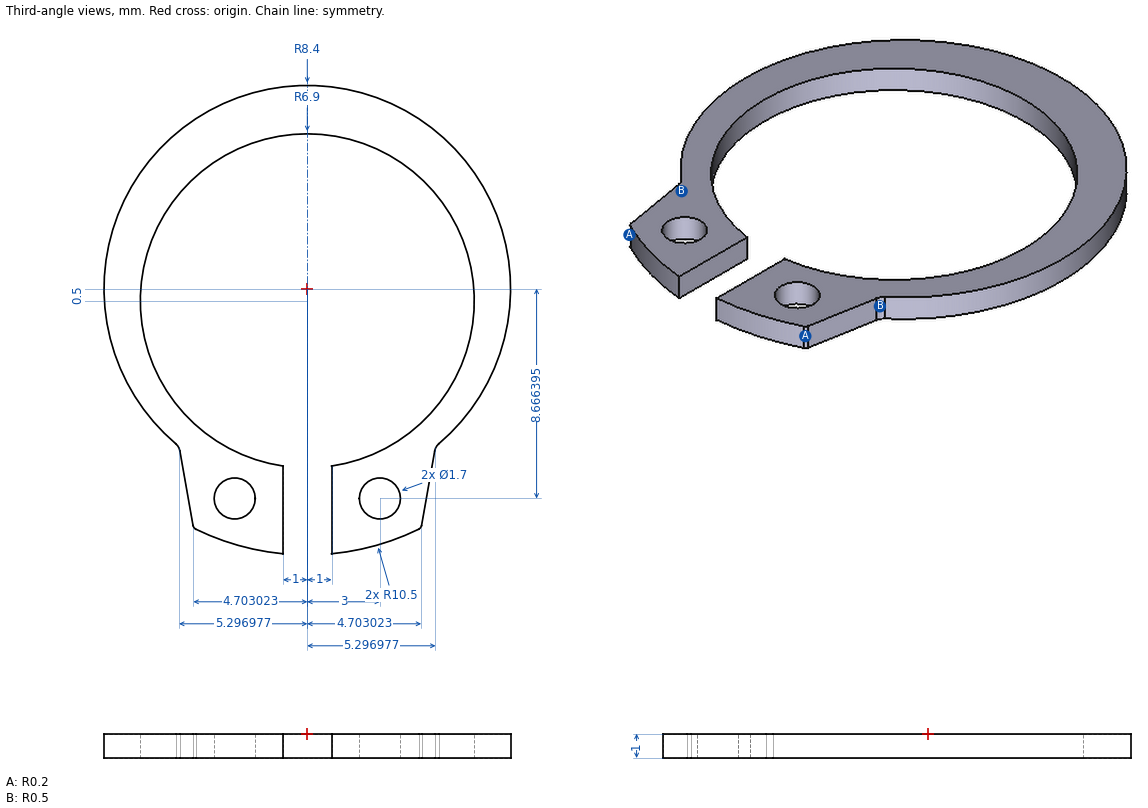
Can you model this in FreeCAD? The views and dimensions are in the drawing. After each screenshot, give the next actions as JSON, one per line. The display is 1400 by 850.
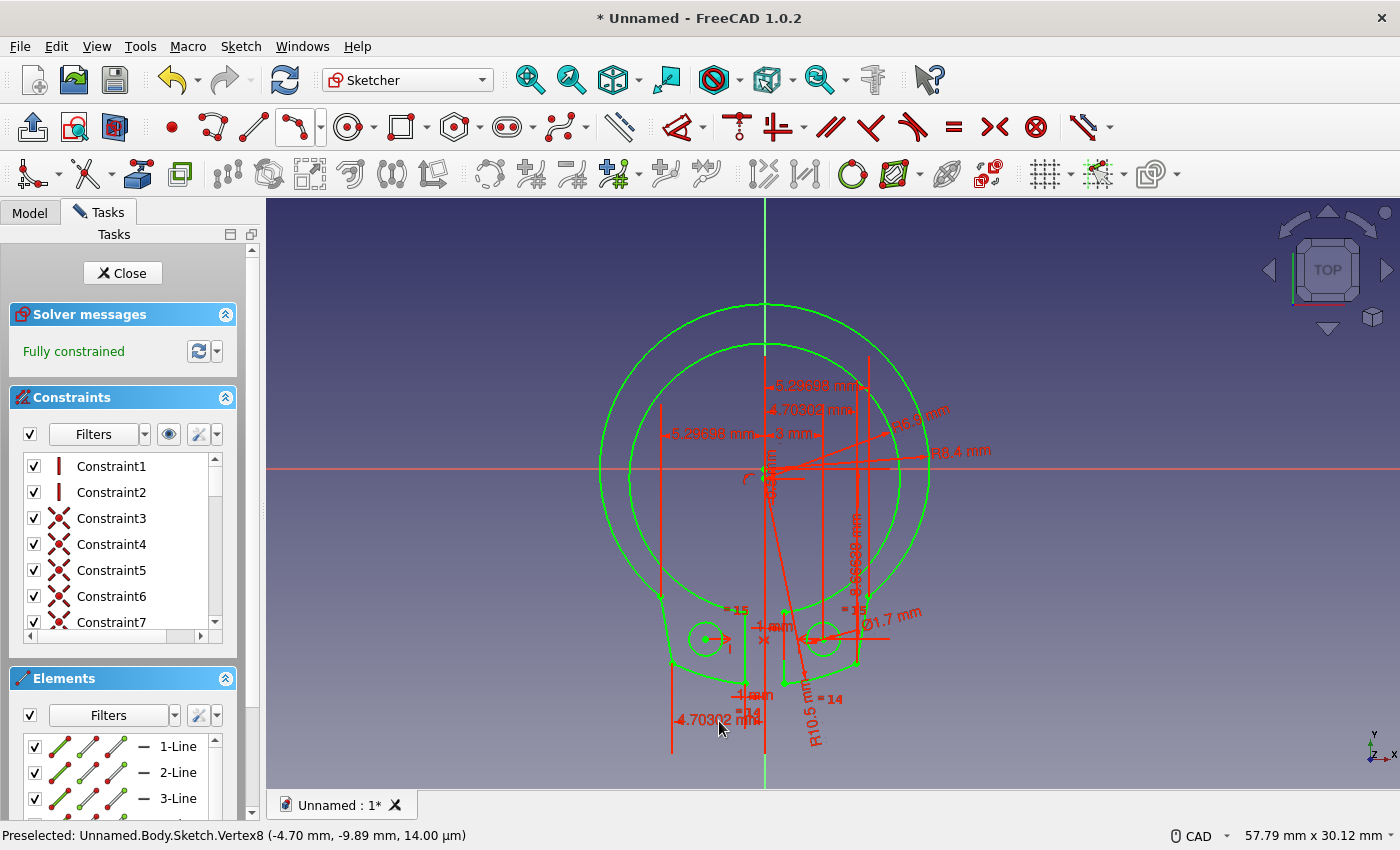
{"action": "left_click", "coordinate": [123, 273]}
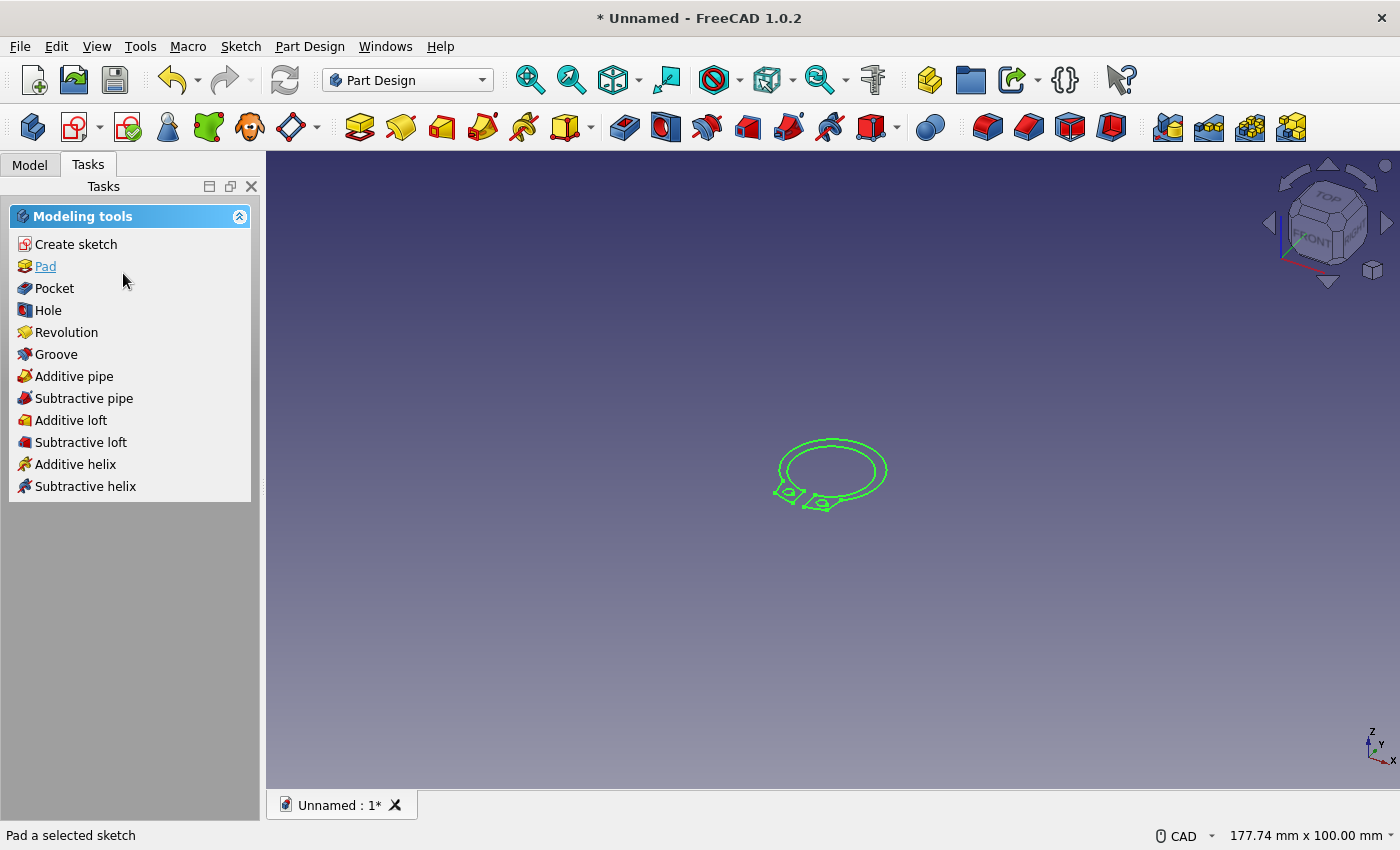
{"action": "left_click", "coordinate": [360, 128]}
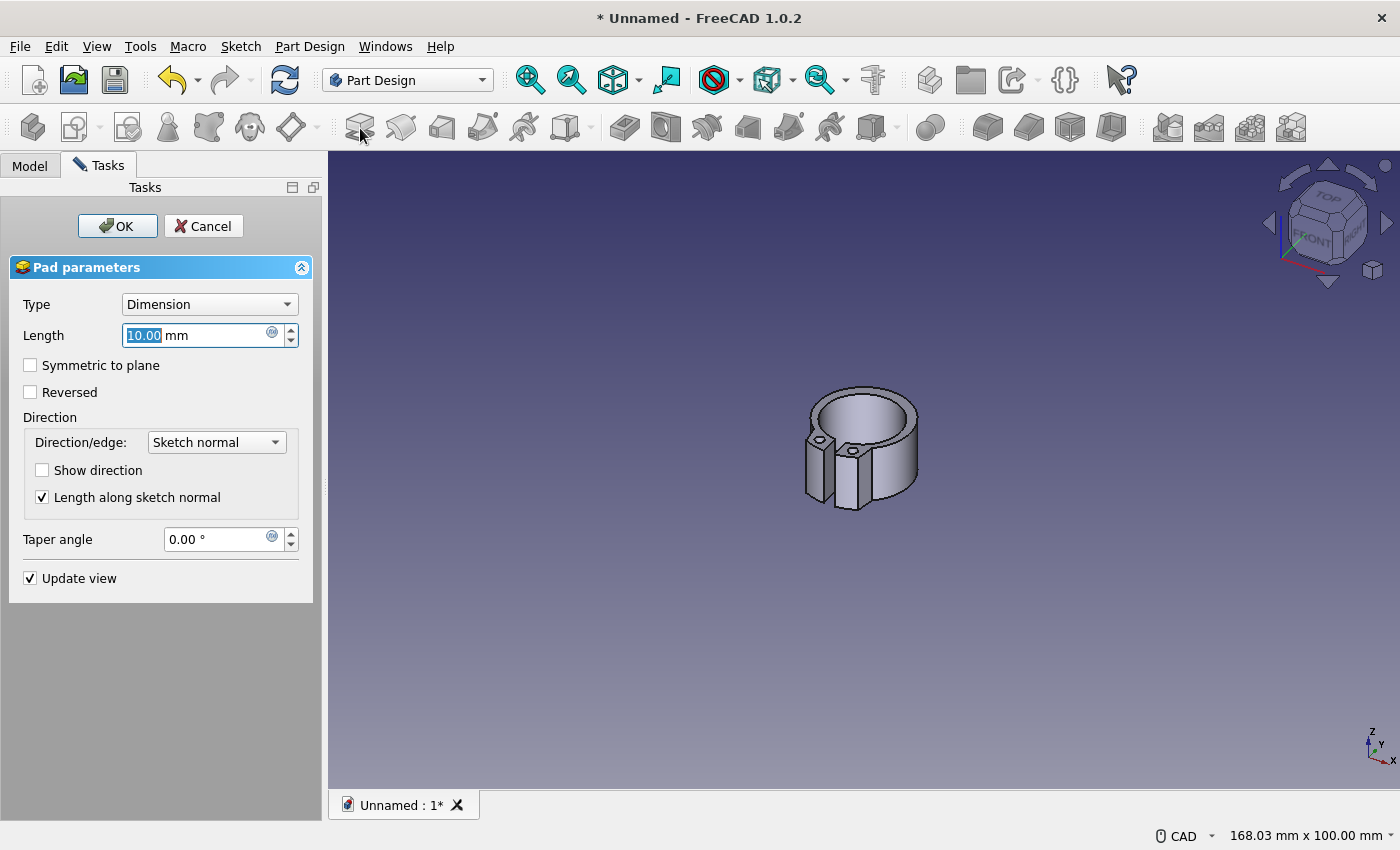
{"action": "type", "text": "1"}
{"action": "key", "text": "Tab"}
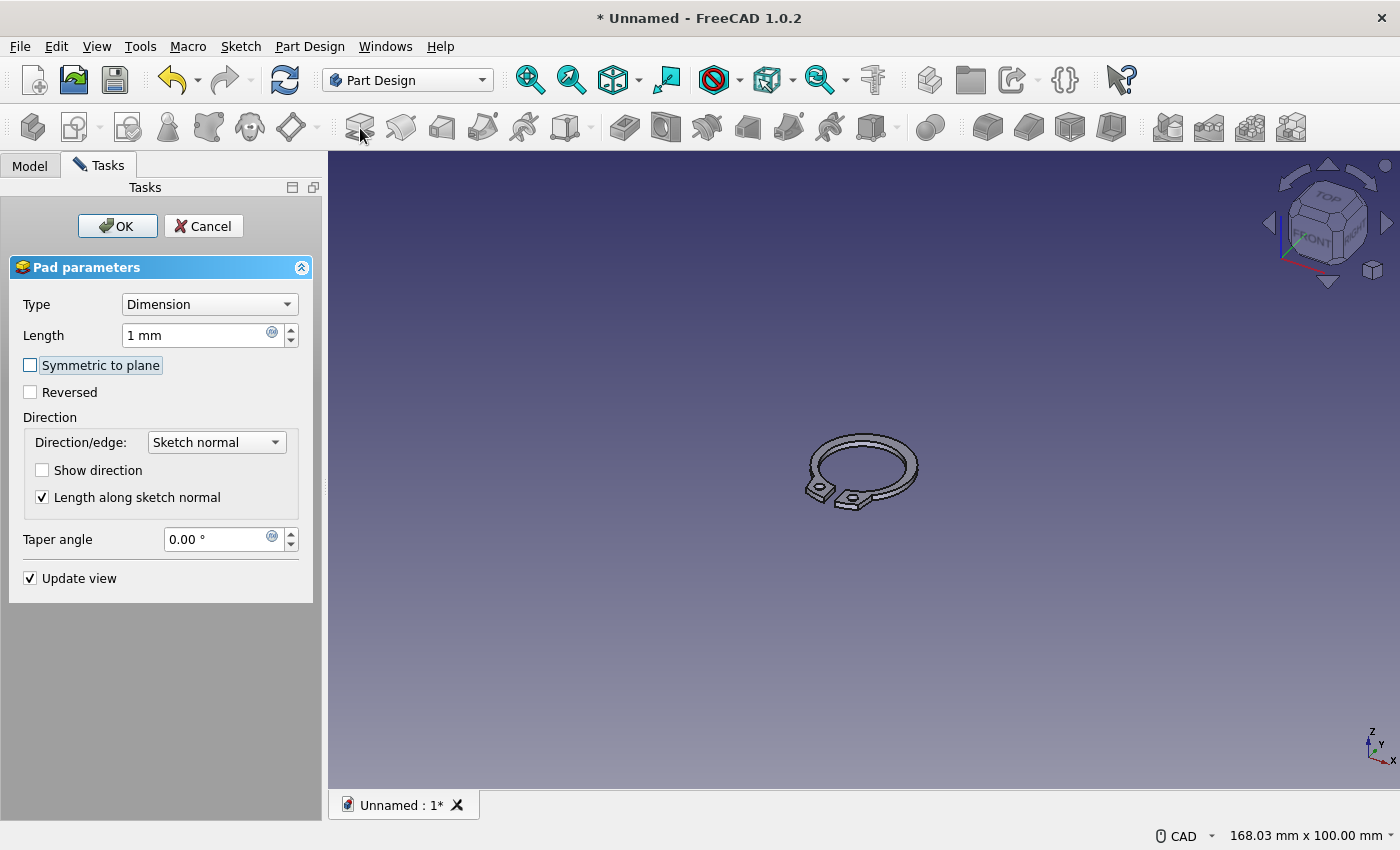
{"action": "left_click", "coordinate": [31, 392]}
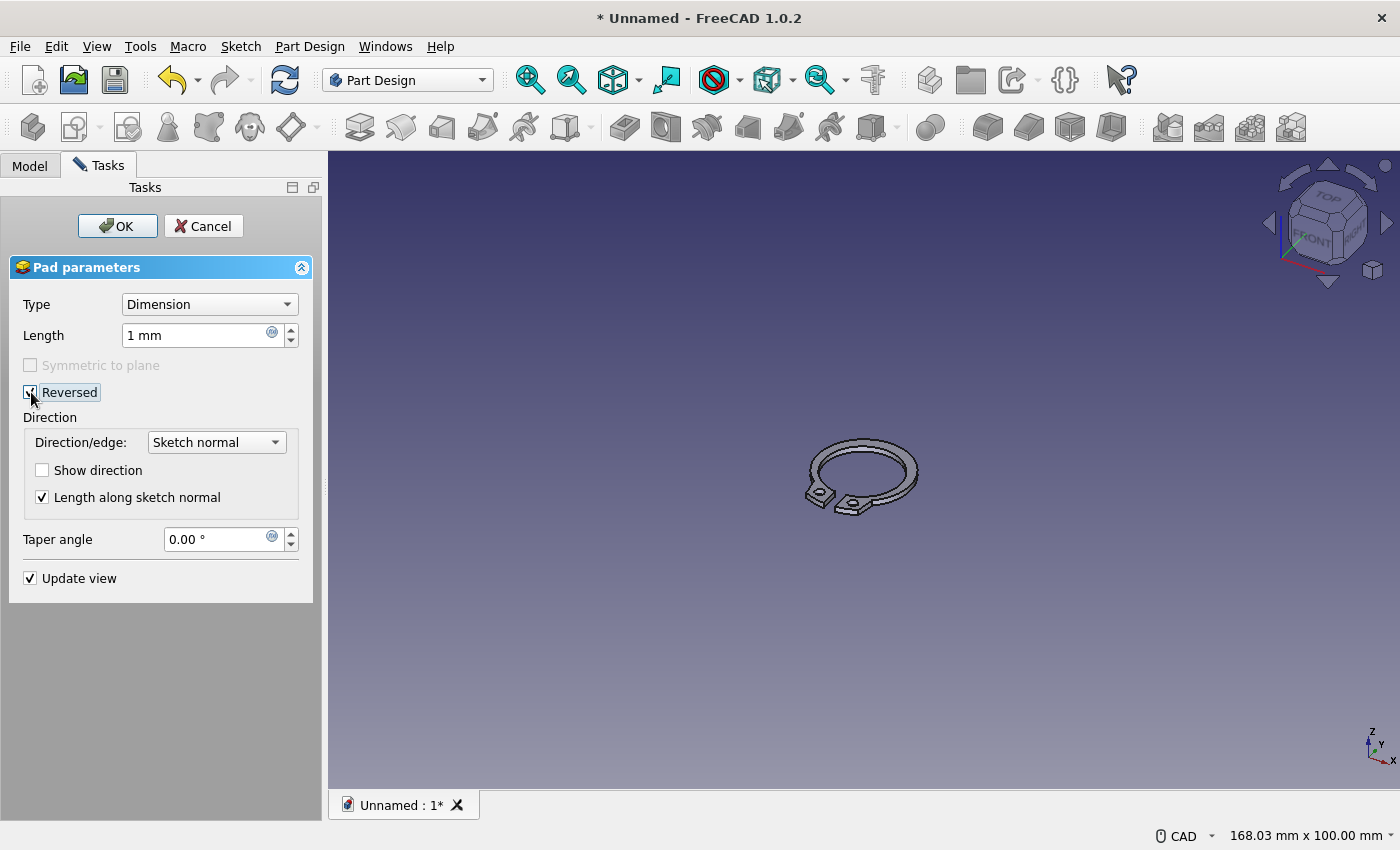
{"action": "left_click", "coordinate": [118, 226]}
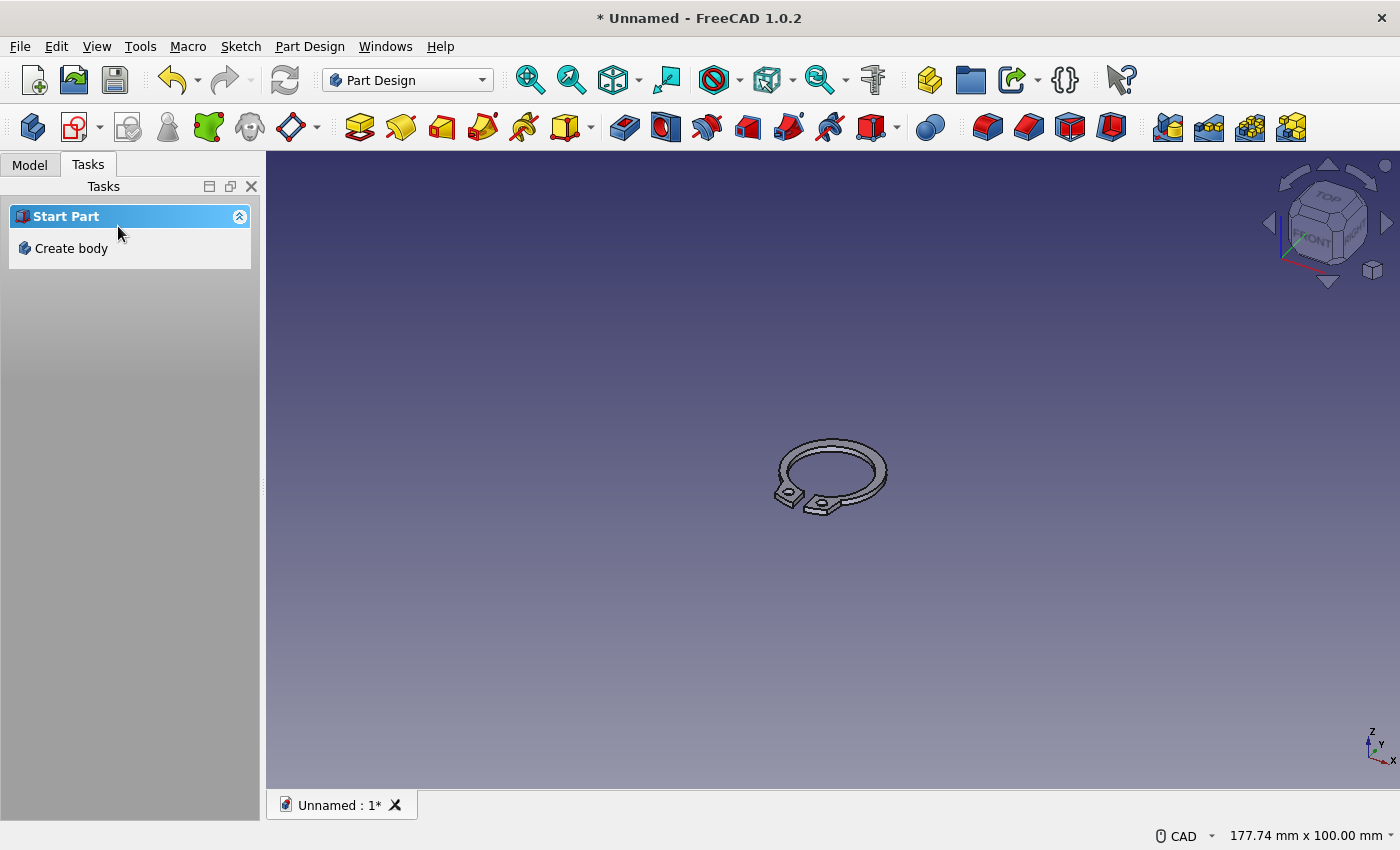
{"action": "left_click", "coordinate": [531, 80]}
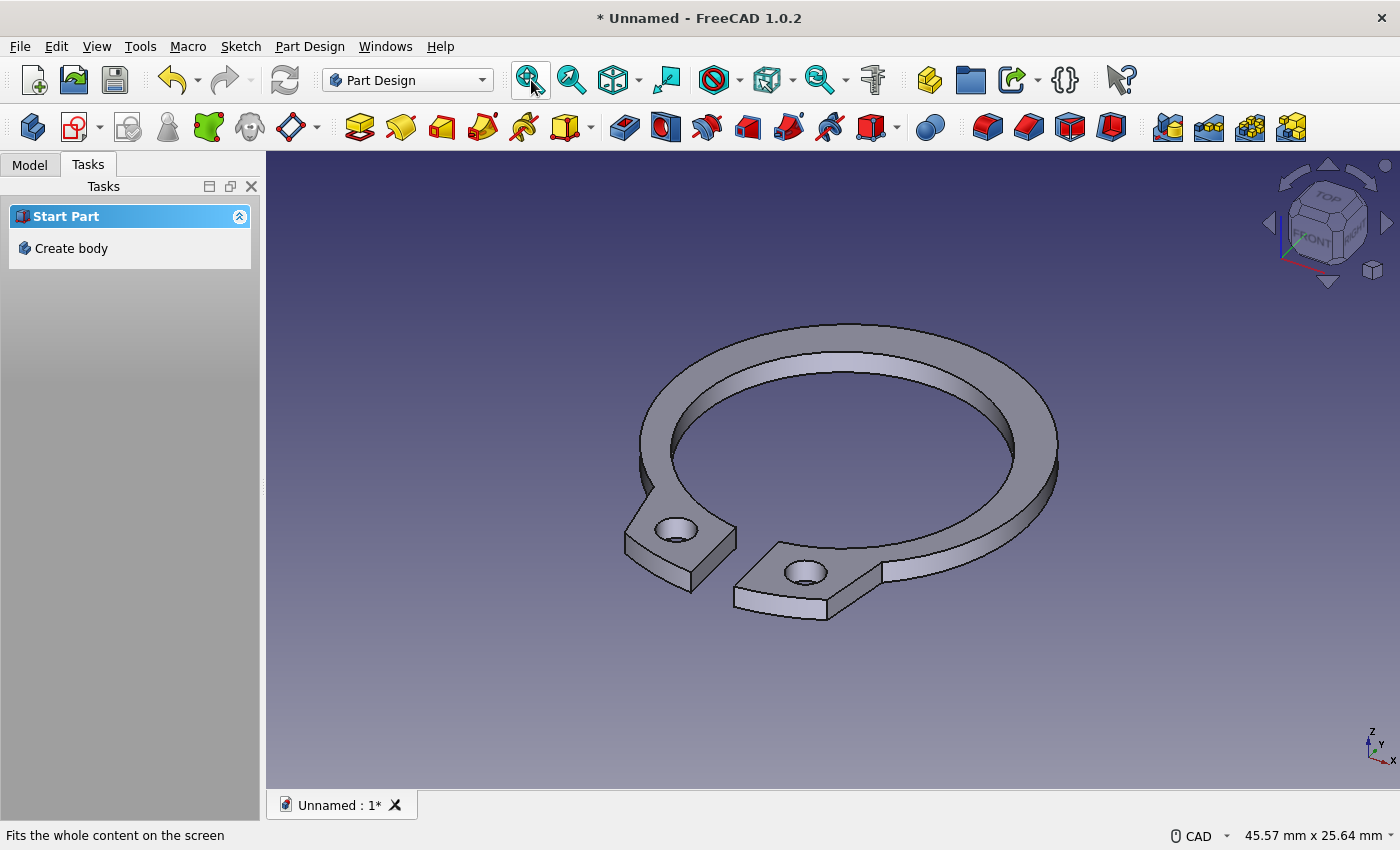
{"action": "left_click", "coordinate": [827, 609]}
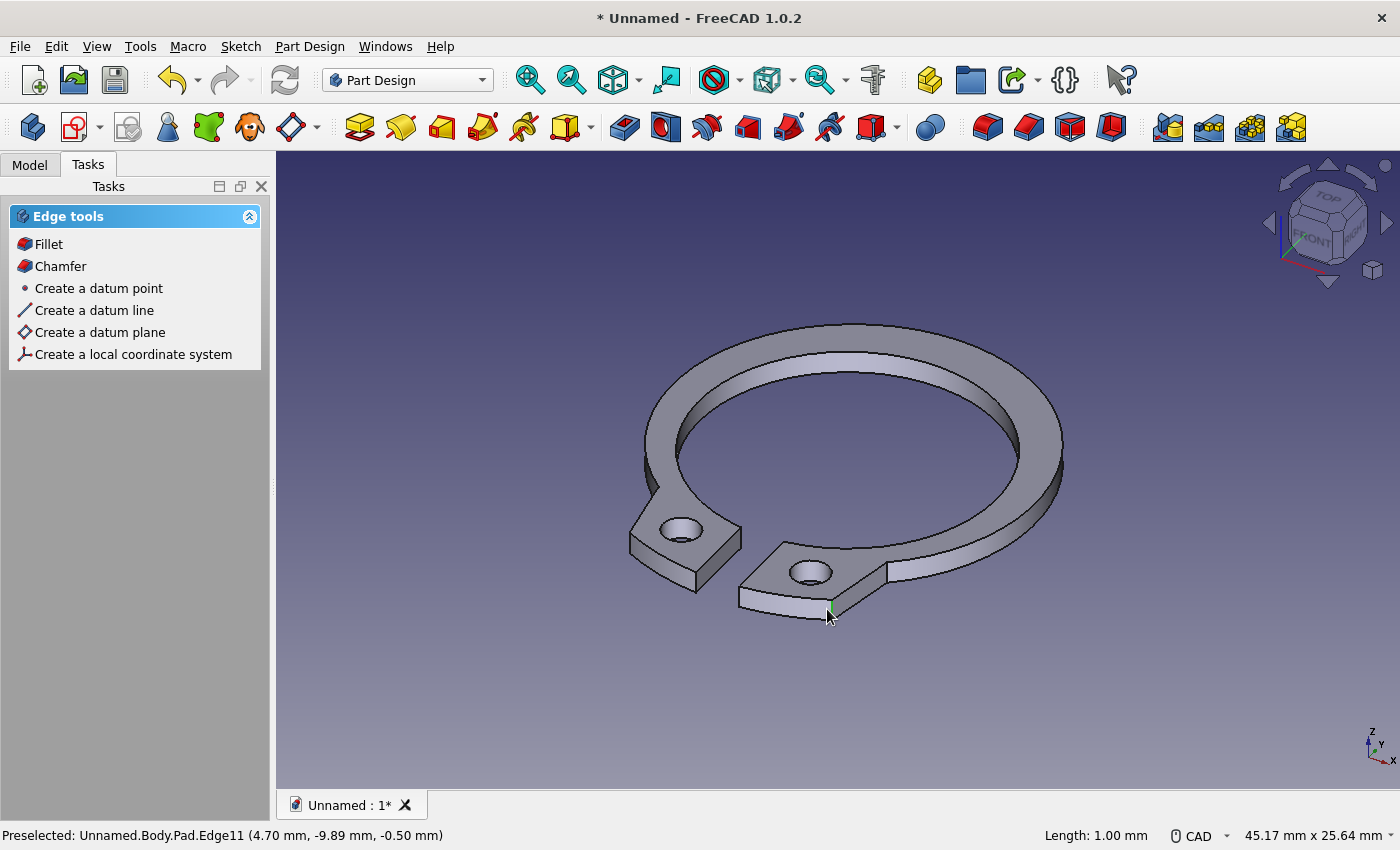
{"action": "key", "text": "0"}